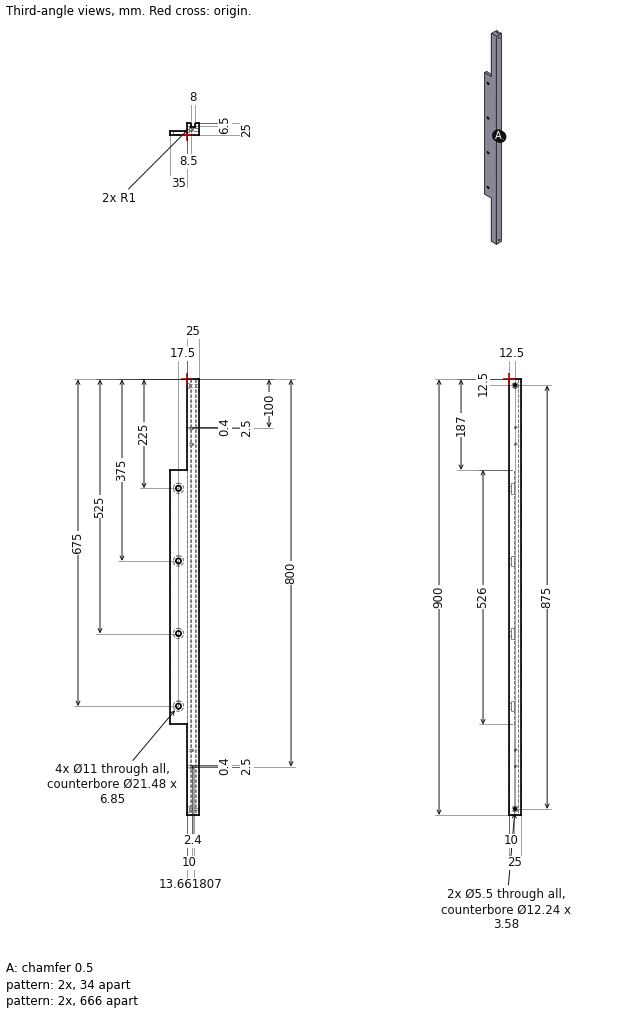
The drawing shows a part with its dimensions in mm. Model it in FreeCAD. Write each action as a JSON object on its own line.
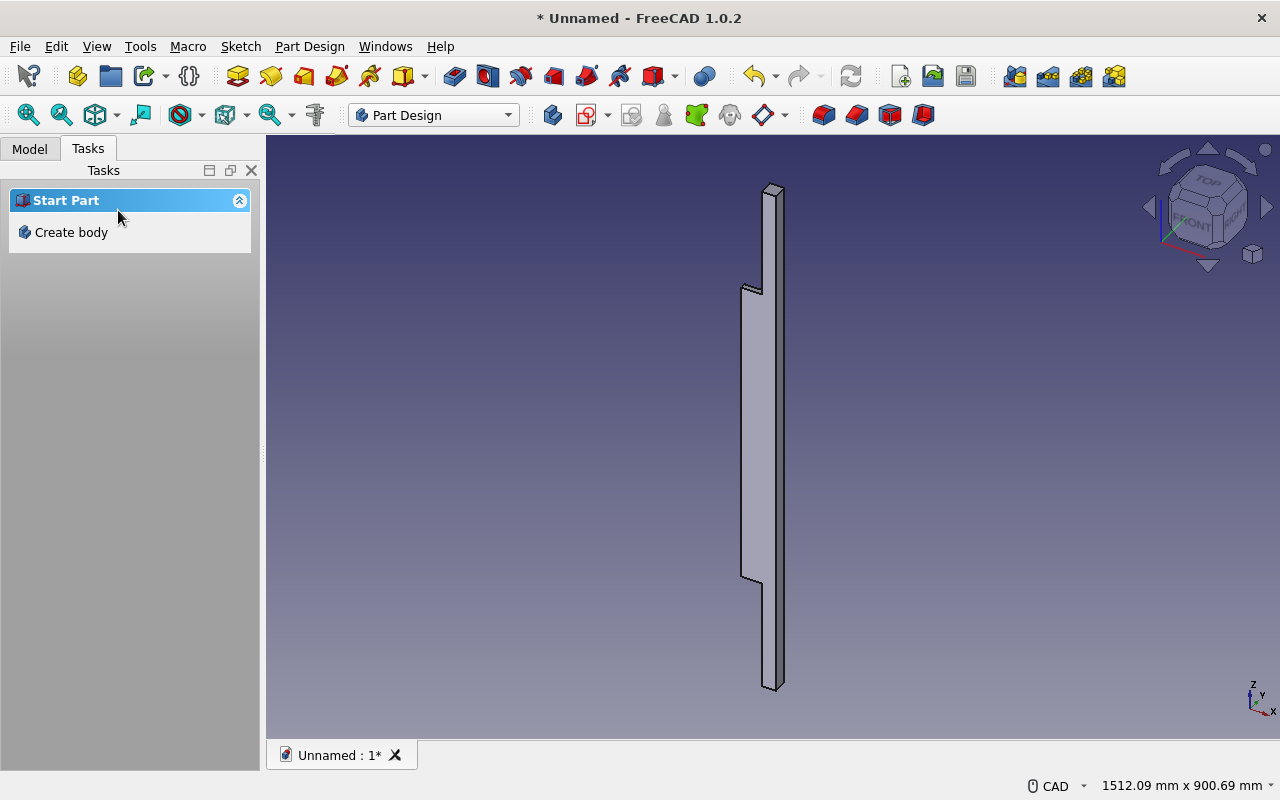
{"action": "key", "text": "0"}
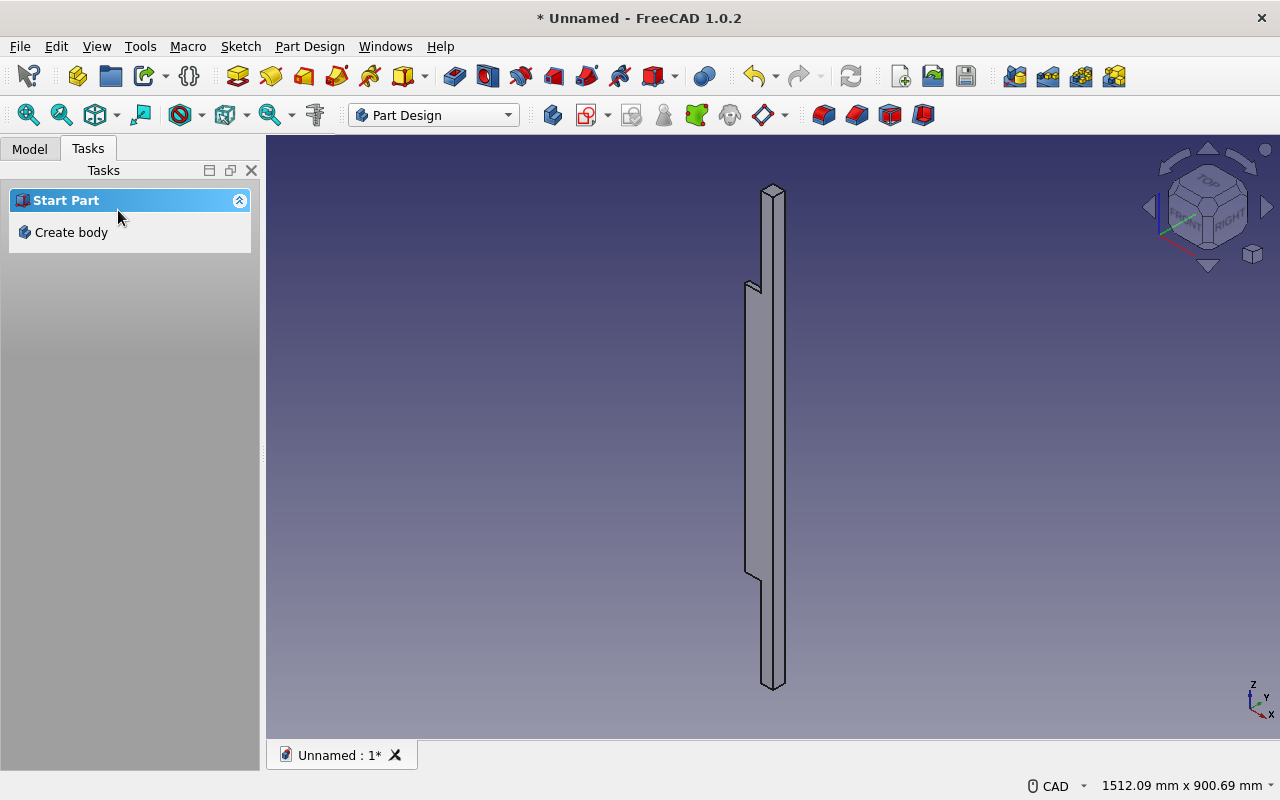
{"action": "key", "text": "2"}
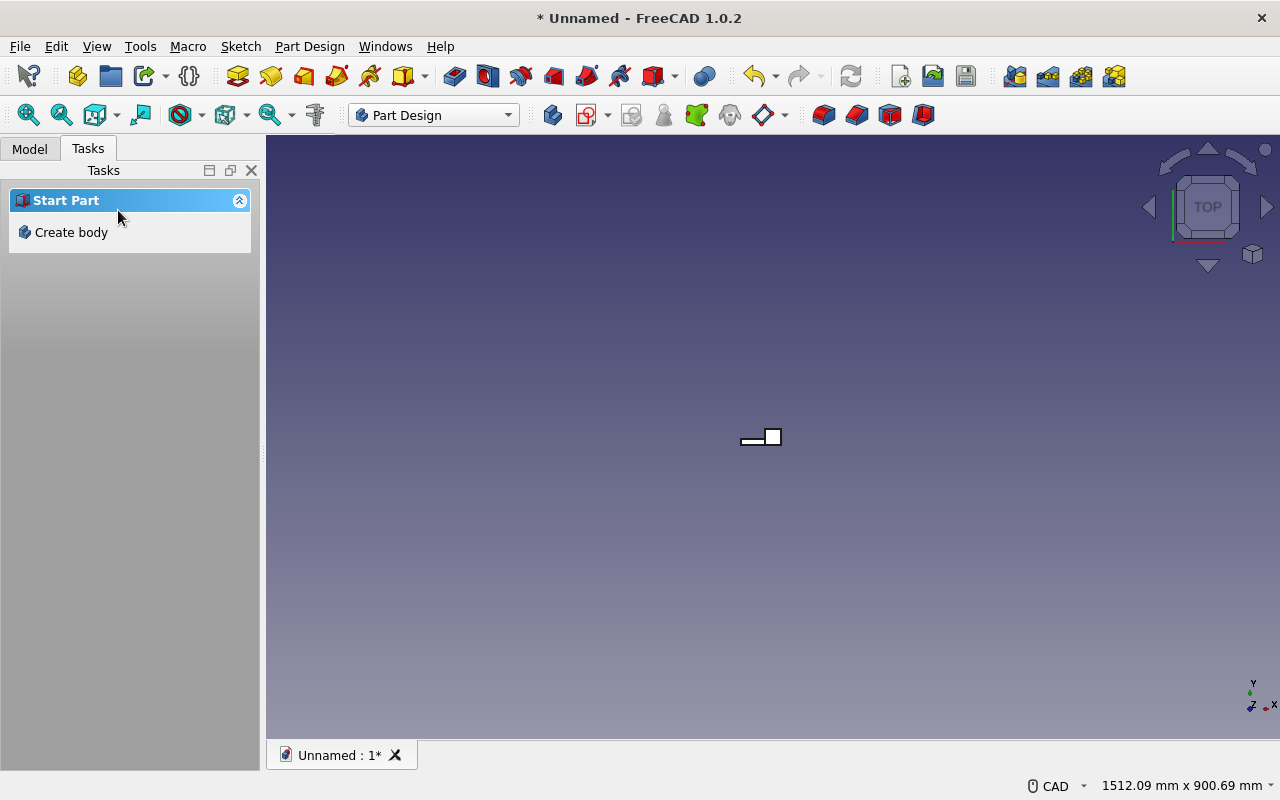
{"action": "left_click", "coordinate": [29, 116]}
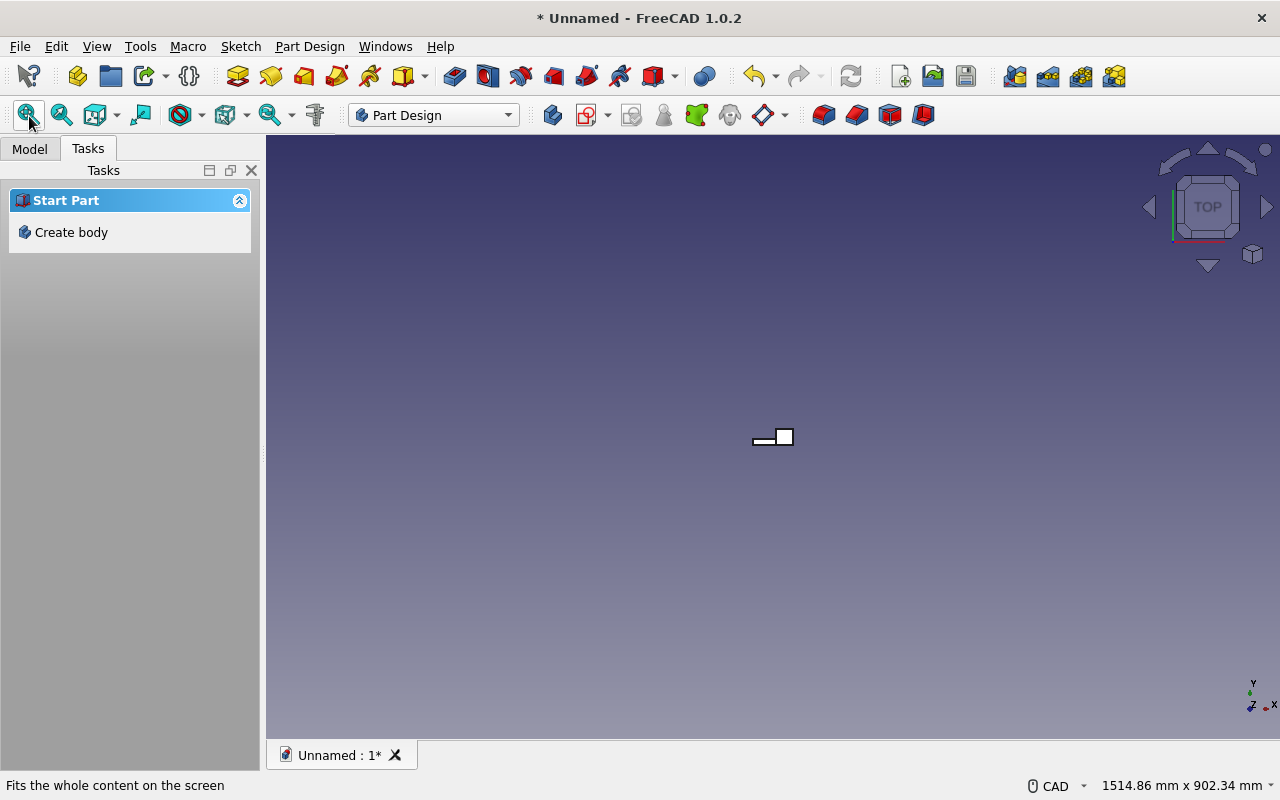
{"action": "left_click", "coordinate": [785, 436]}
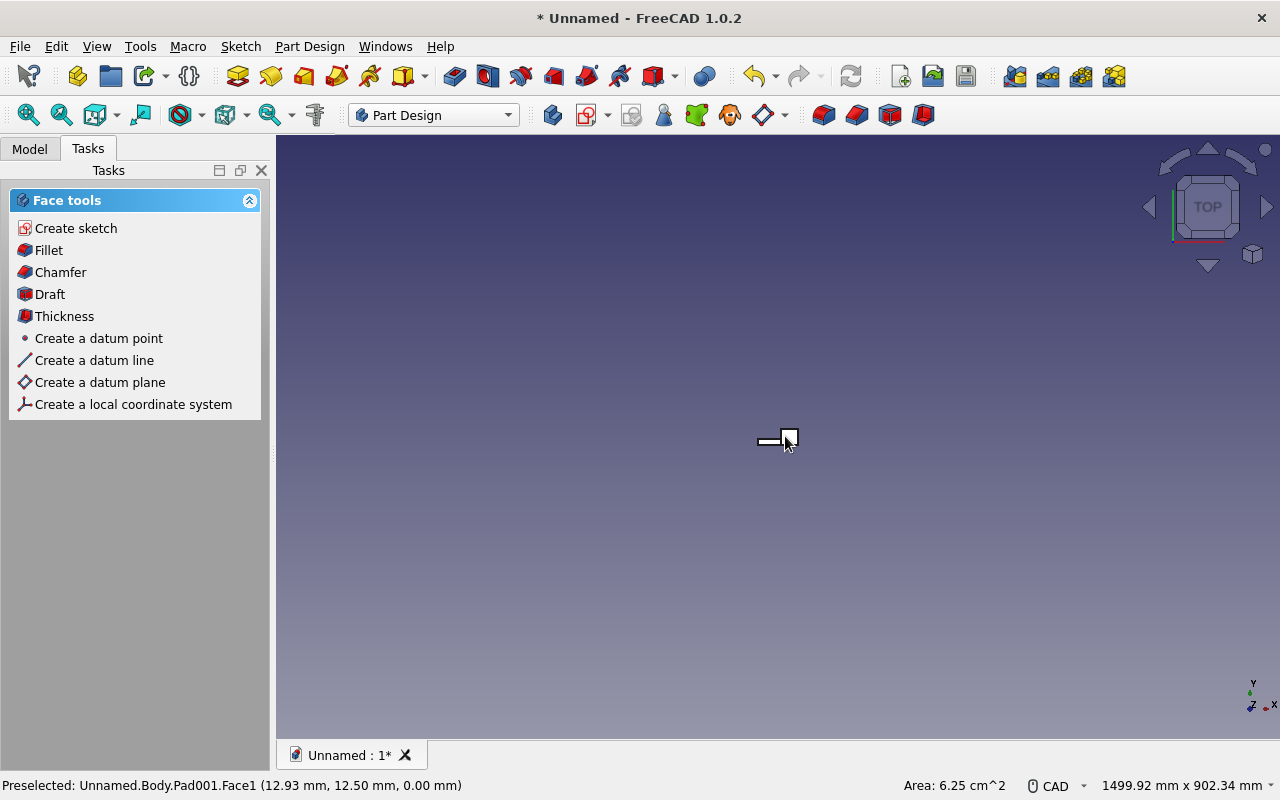
{"action": "left_click", "coordinate": [586, 116]}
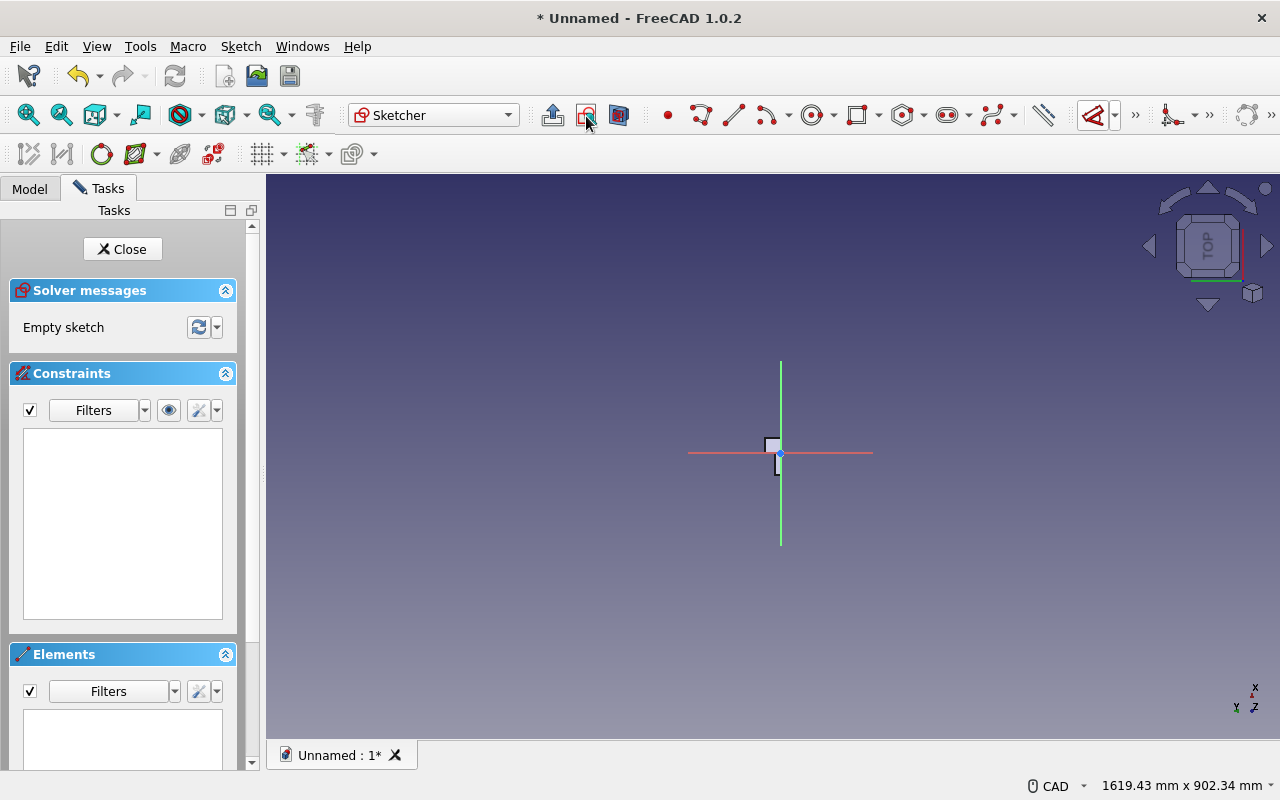
{"action": "scroll", "coordinate": [771, 445], "scroll_direction": "up", "scroll_amount": 15}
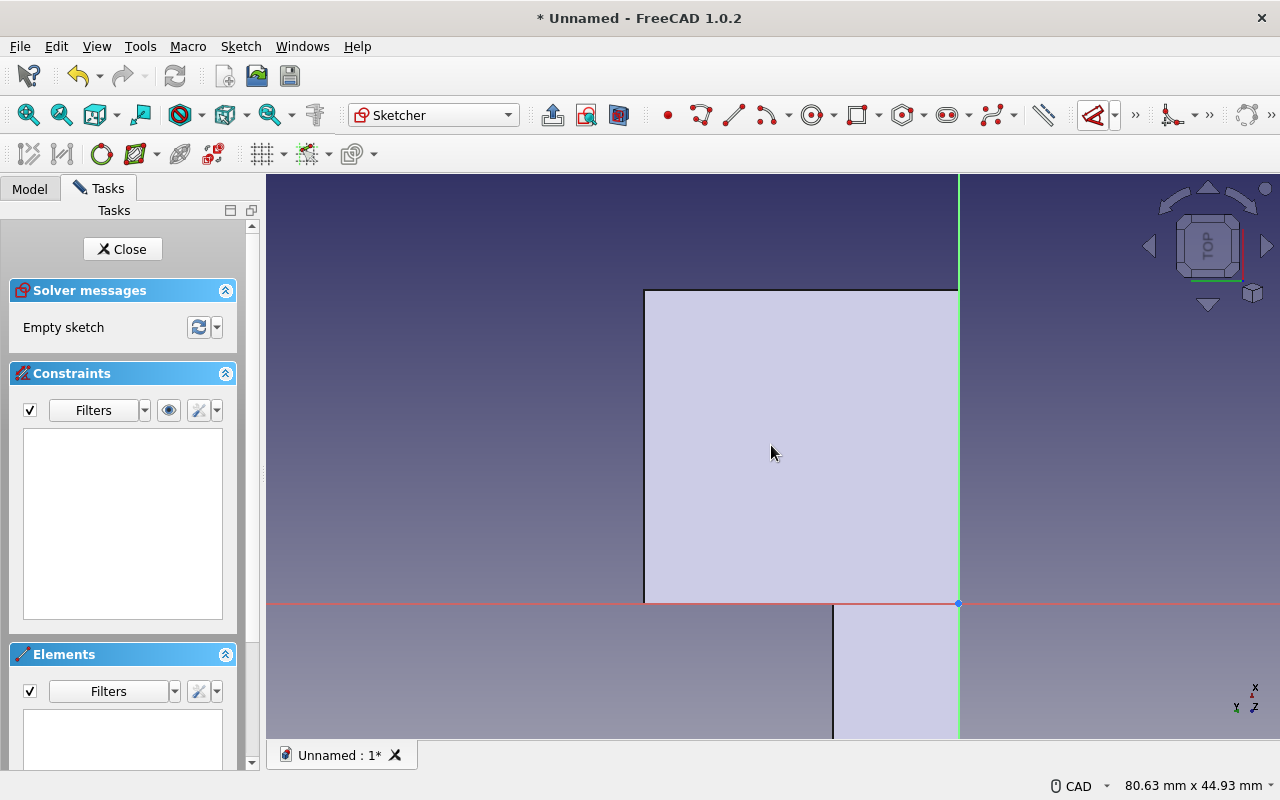
{"action": "scroll", "coordinate": [684, 441], "scroll_direction": "up", "scroll_amount": 5}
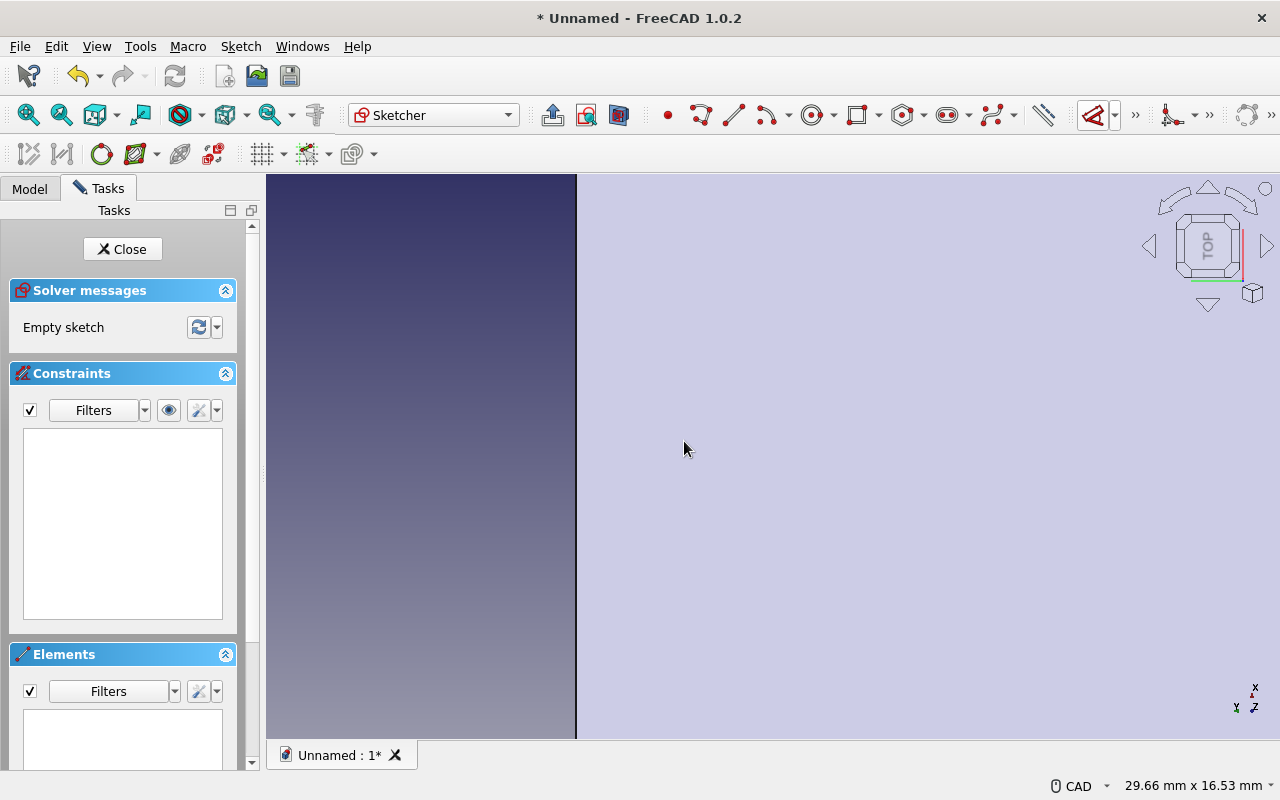
{"action": "left_click", "coordinate": [734, 116]}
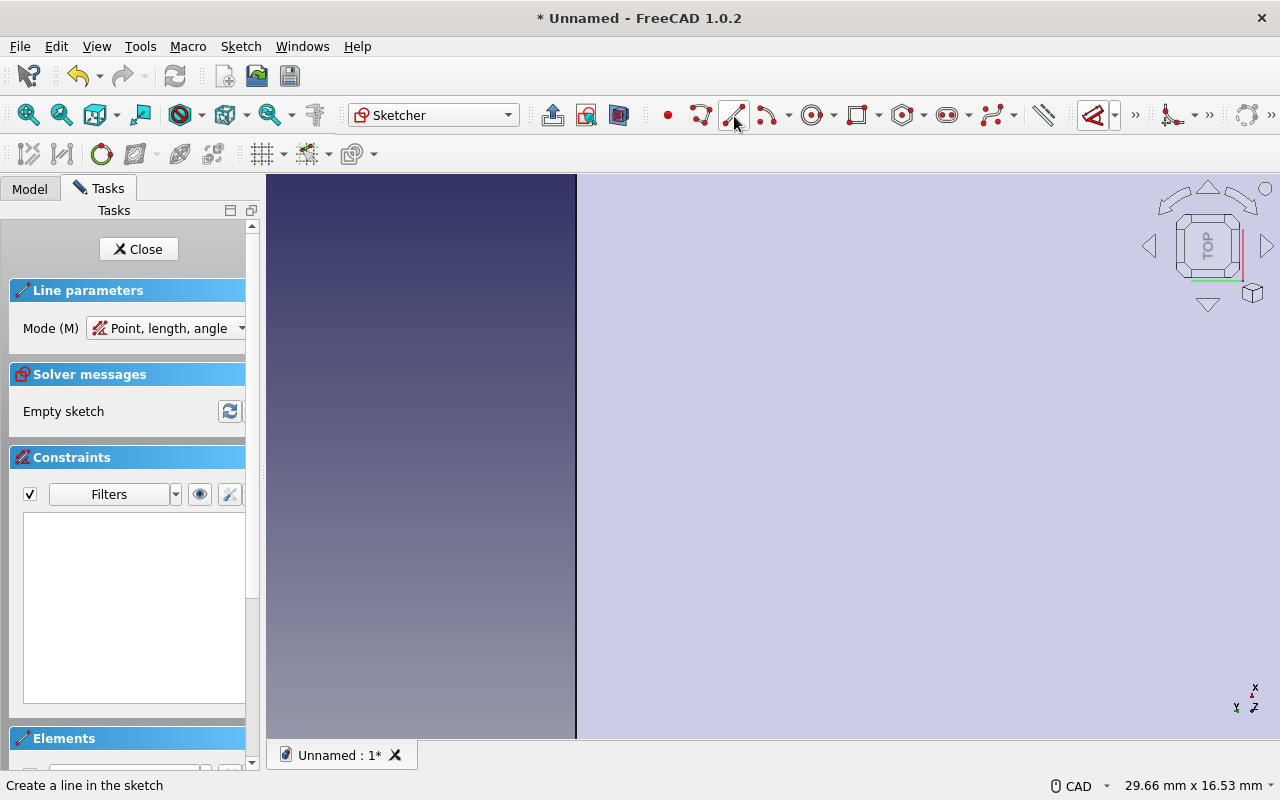
{"action": "left_click", "coordinate": [832, 592]}
{"action": "left_click", "coordinate": [832, 319]}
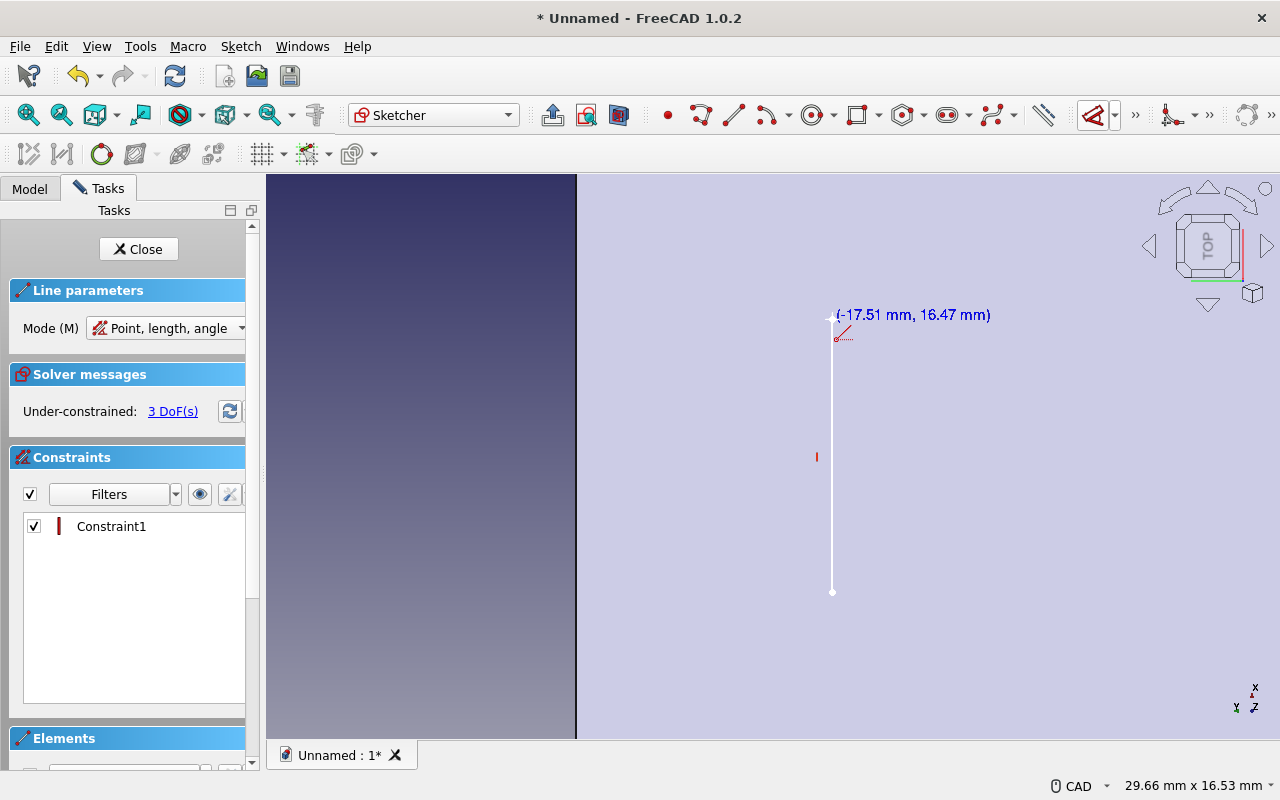
{"action": "key", "text": "g m"}